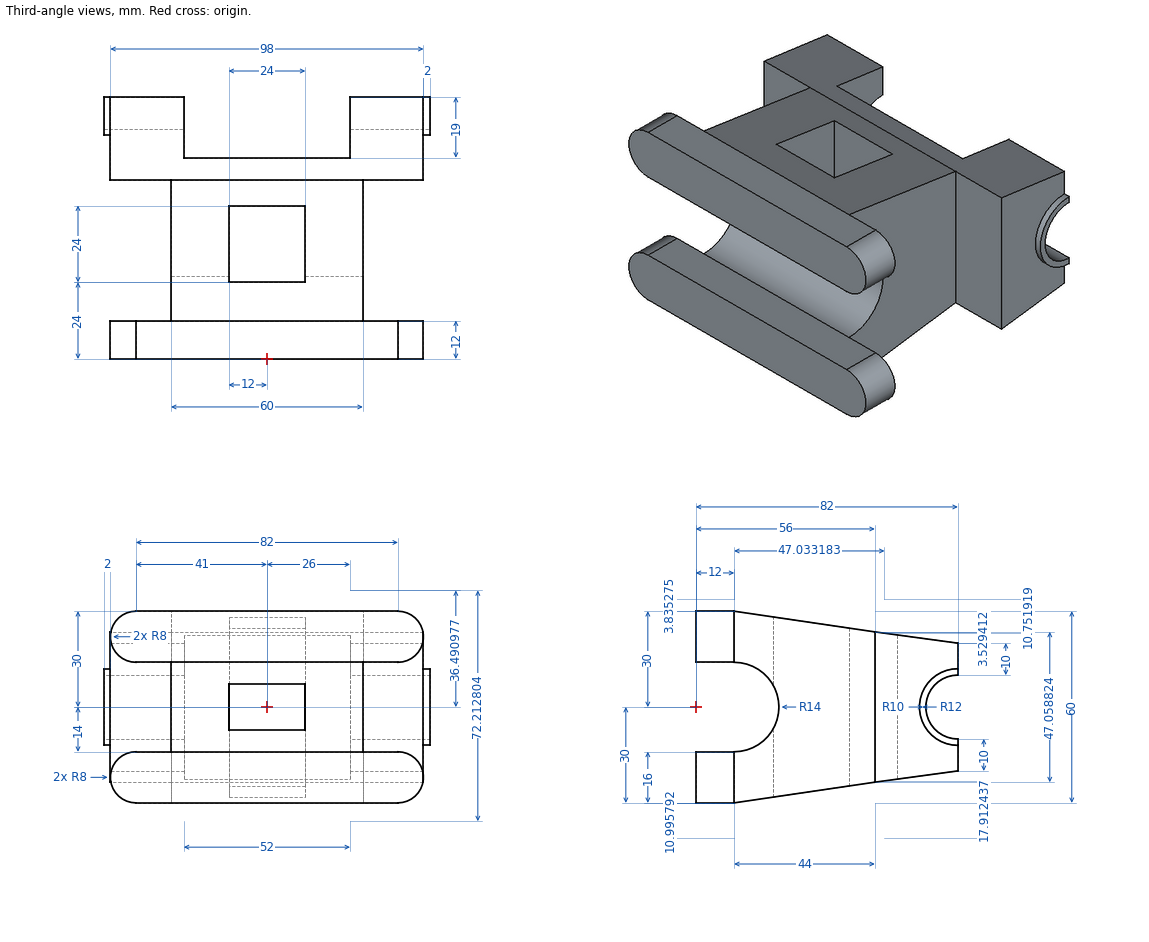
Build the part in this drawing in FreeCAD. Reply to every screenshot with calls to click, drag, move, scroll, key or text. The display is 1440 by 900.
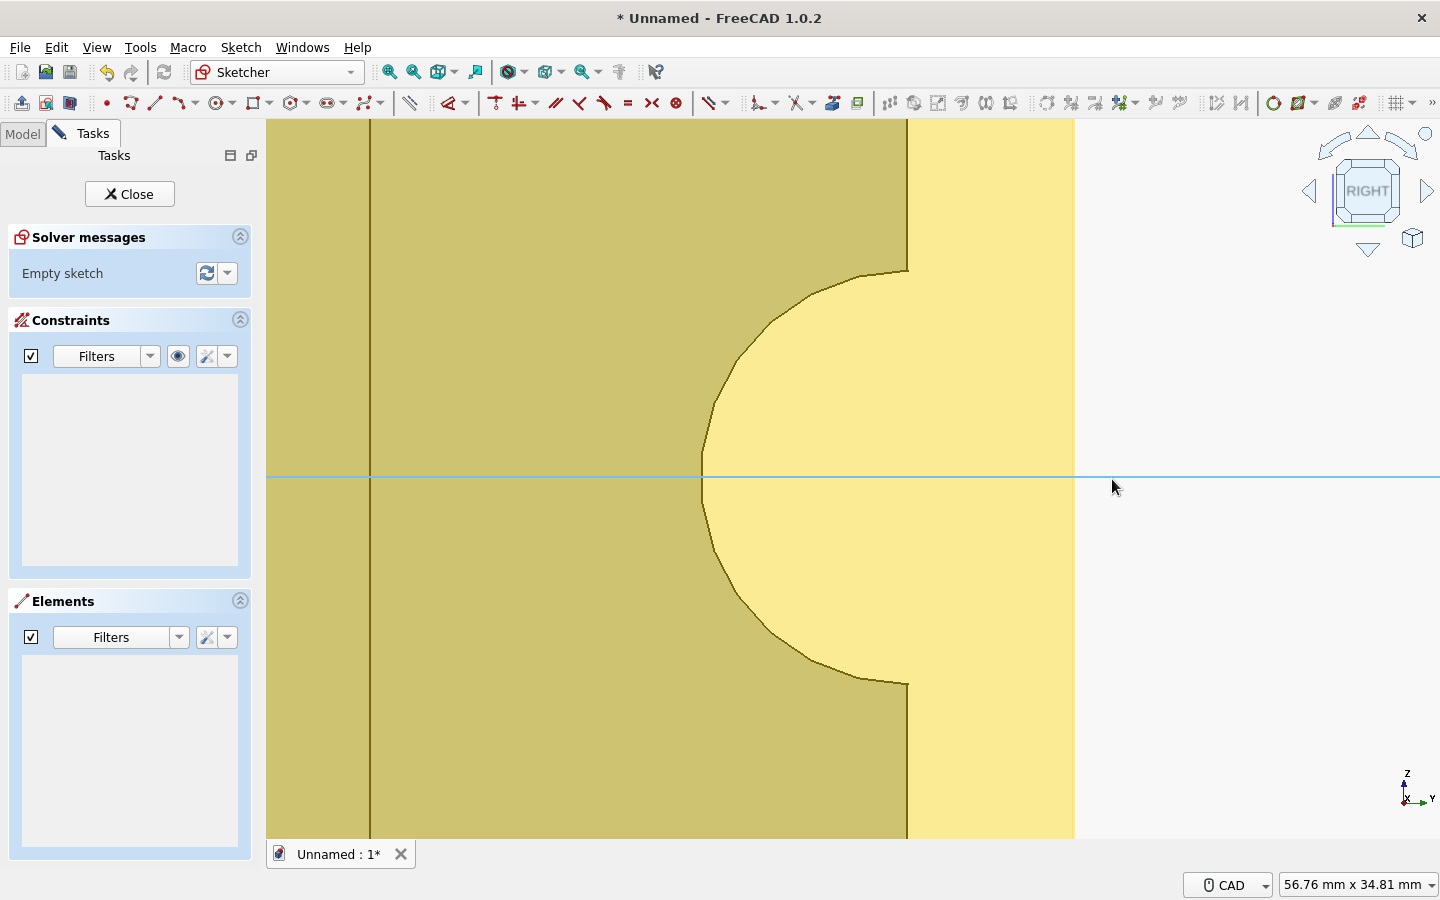
click(156, 104)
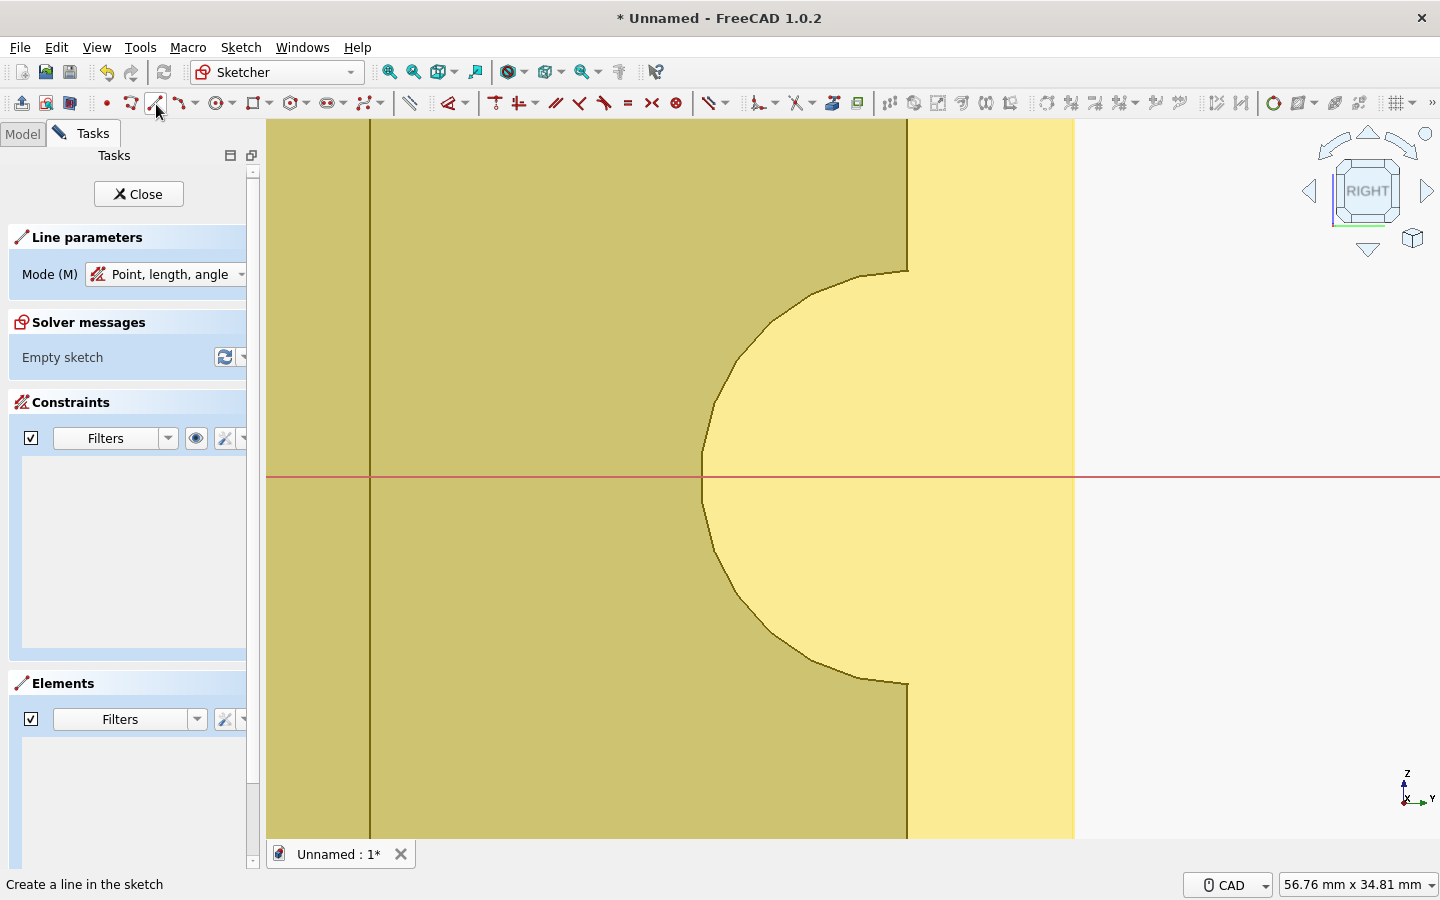
click(908, 271)
click(908, 229)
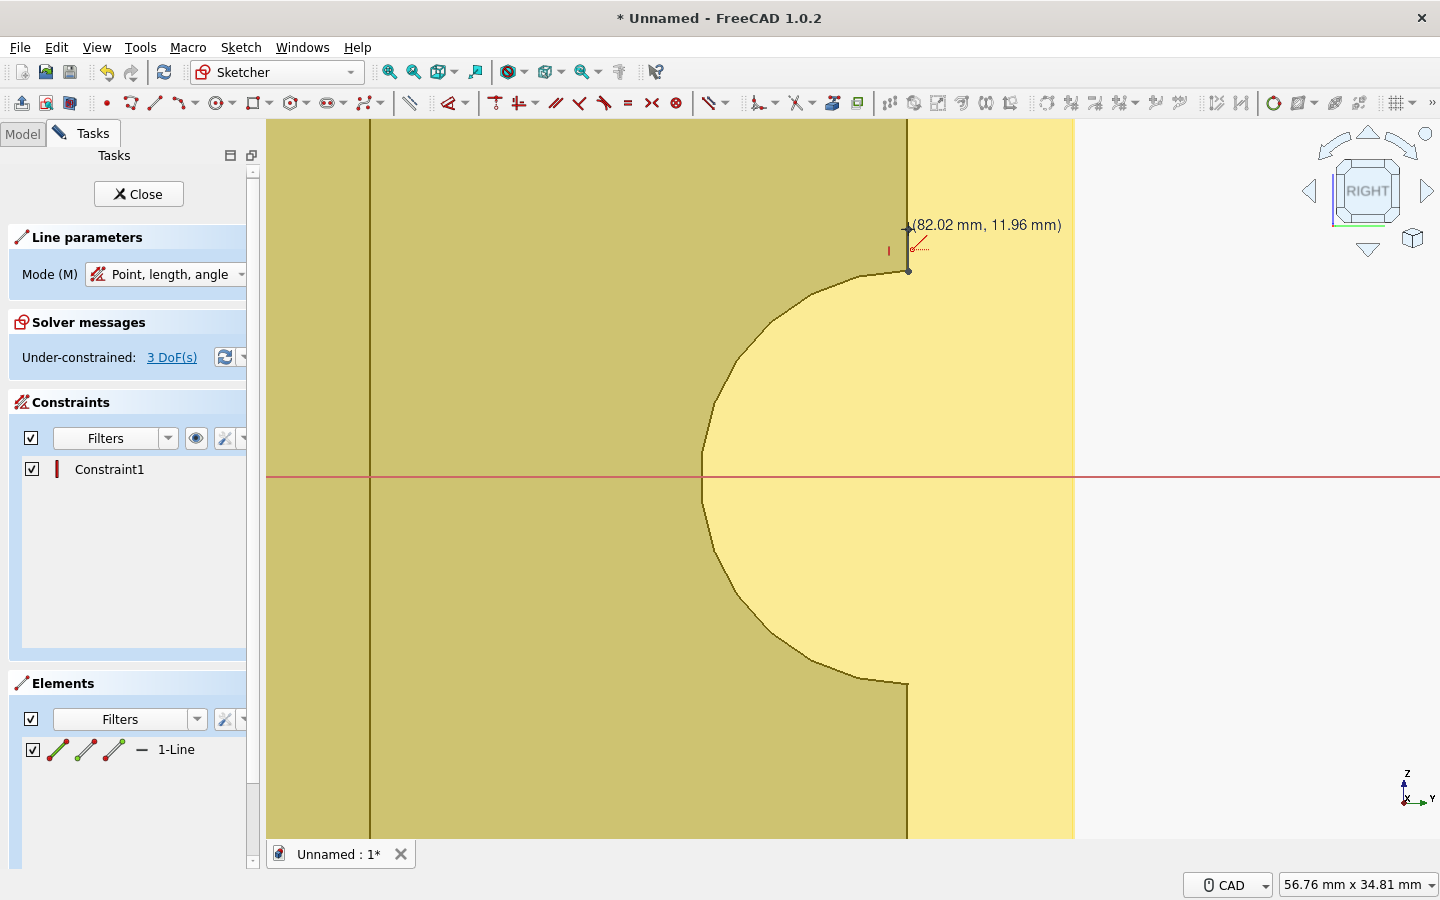
click(908, 726)
click(908, 684)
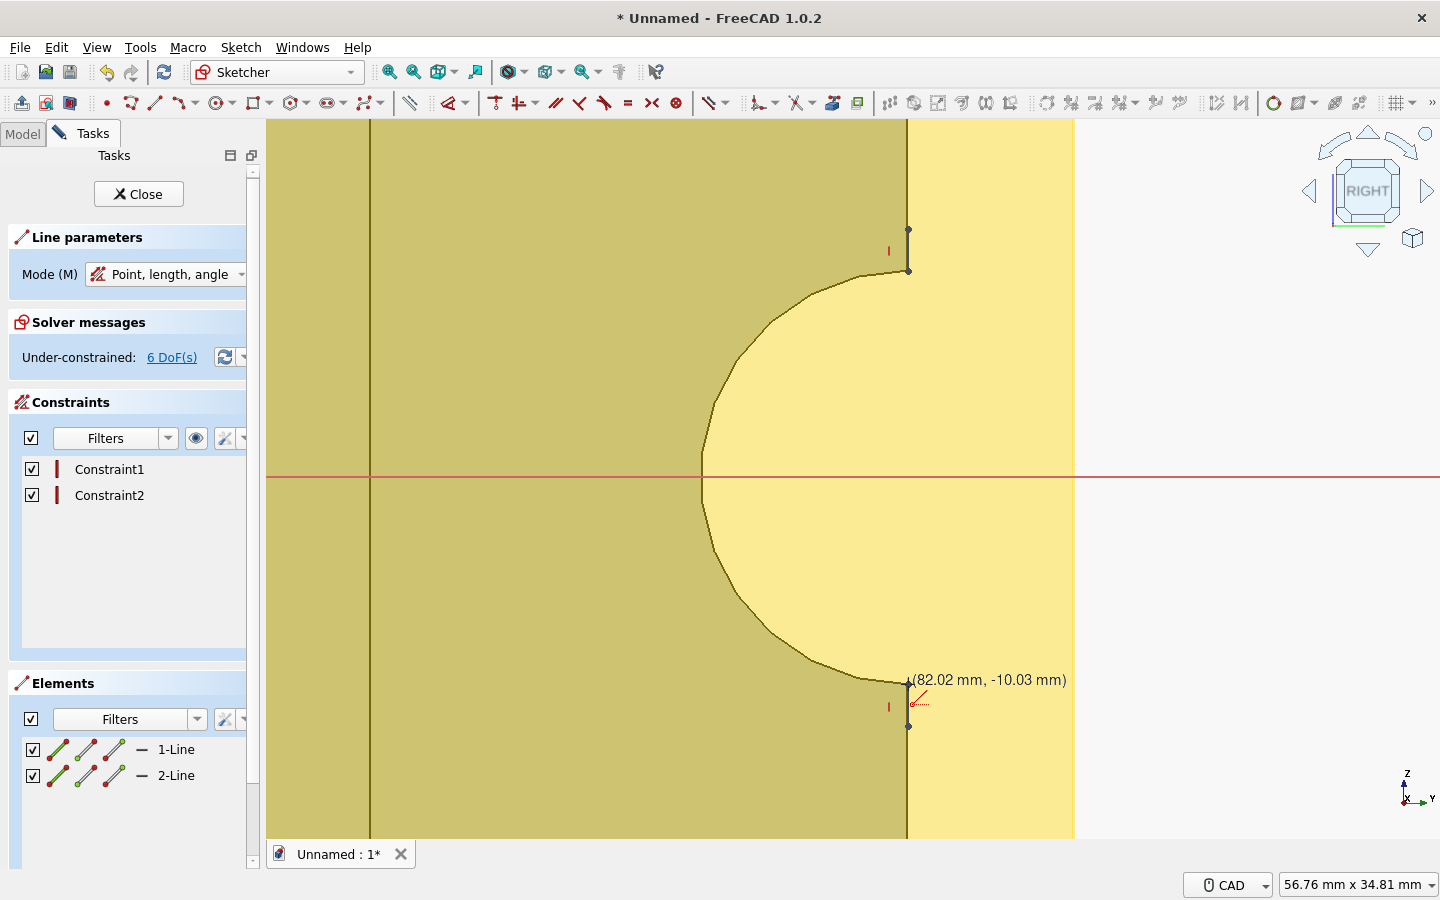
click(180, 104)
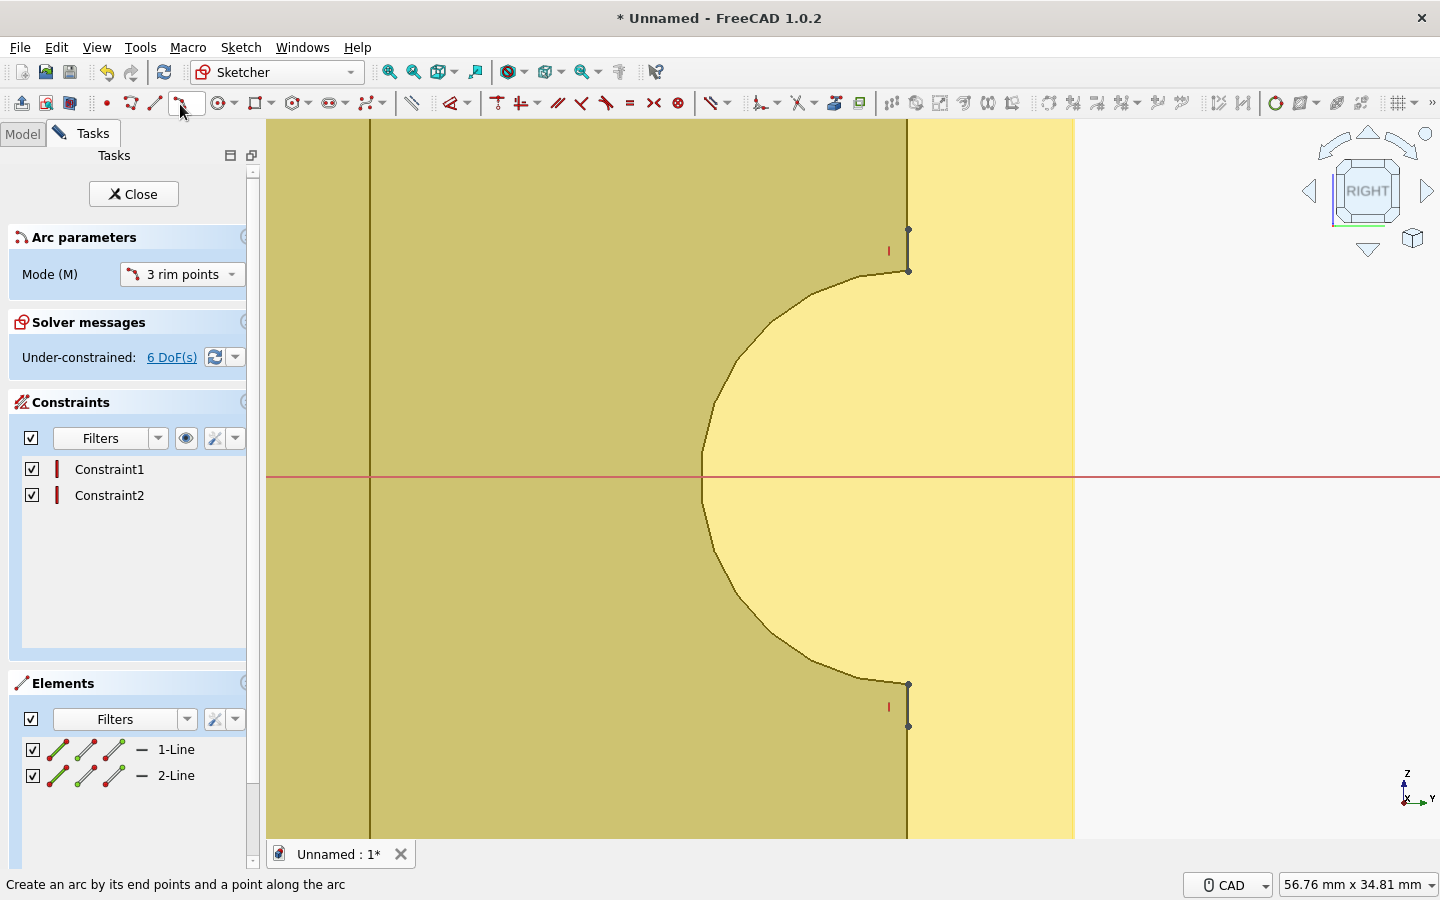
click(908, 230)
click(908, 727)
click(671, 401)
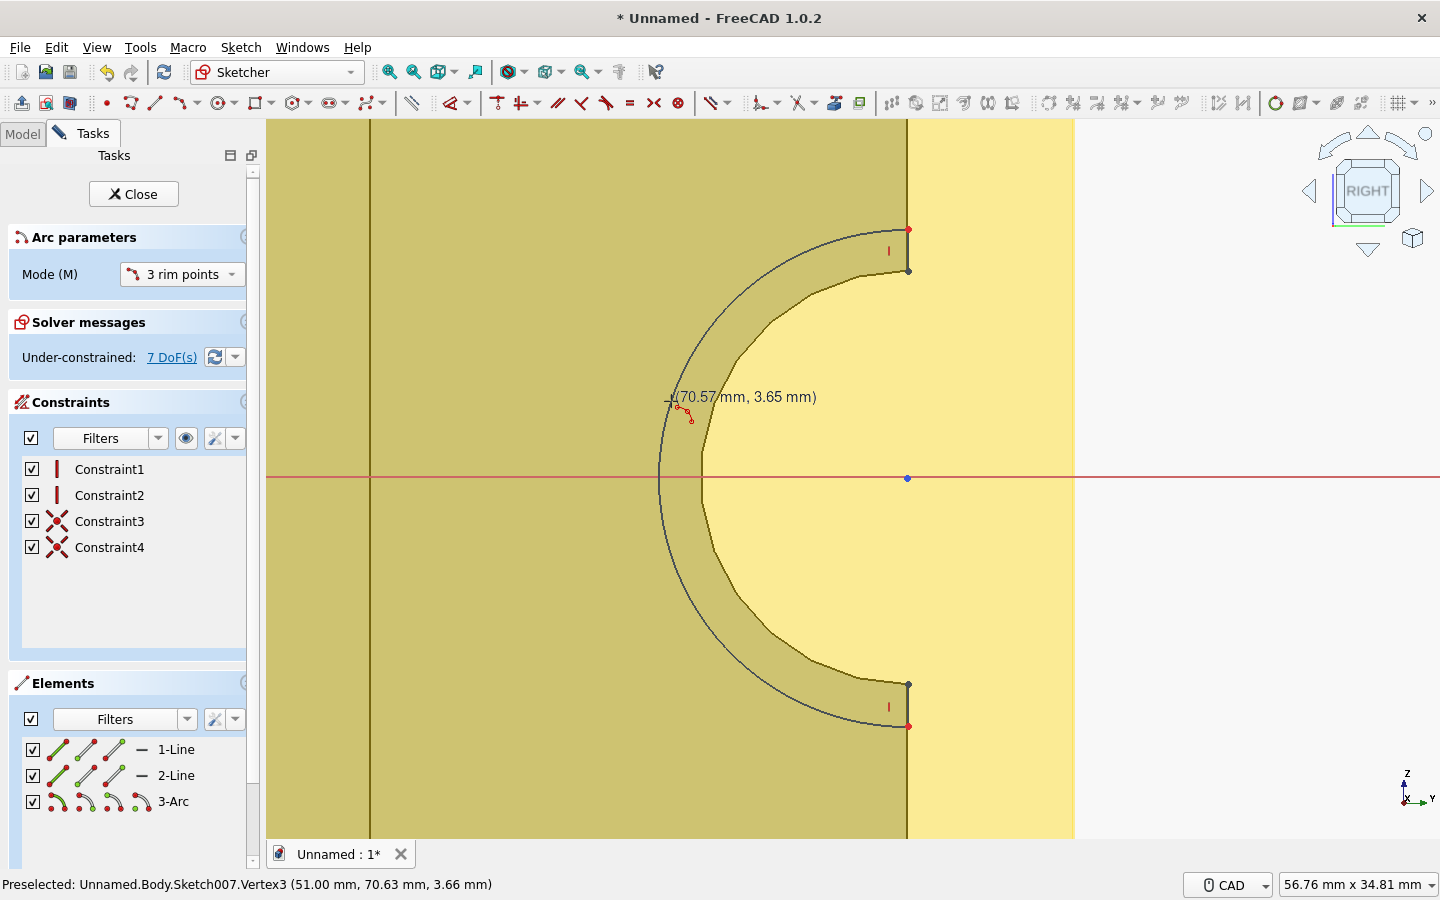
click(908, 685)
click(908, 272)
click(711, 414)
key(Escape)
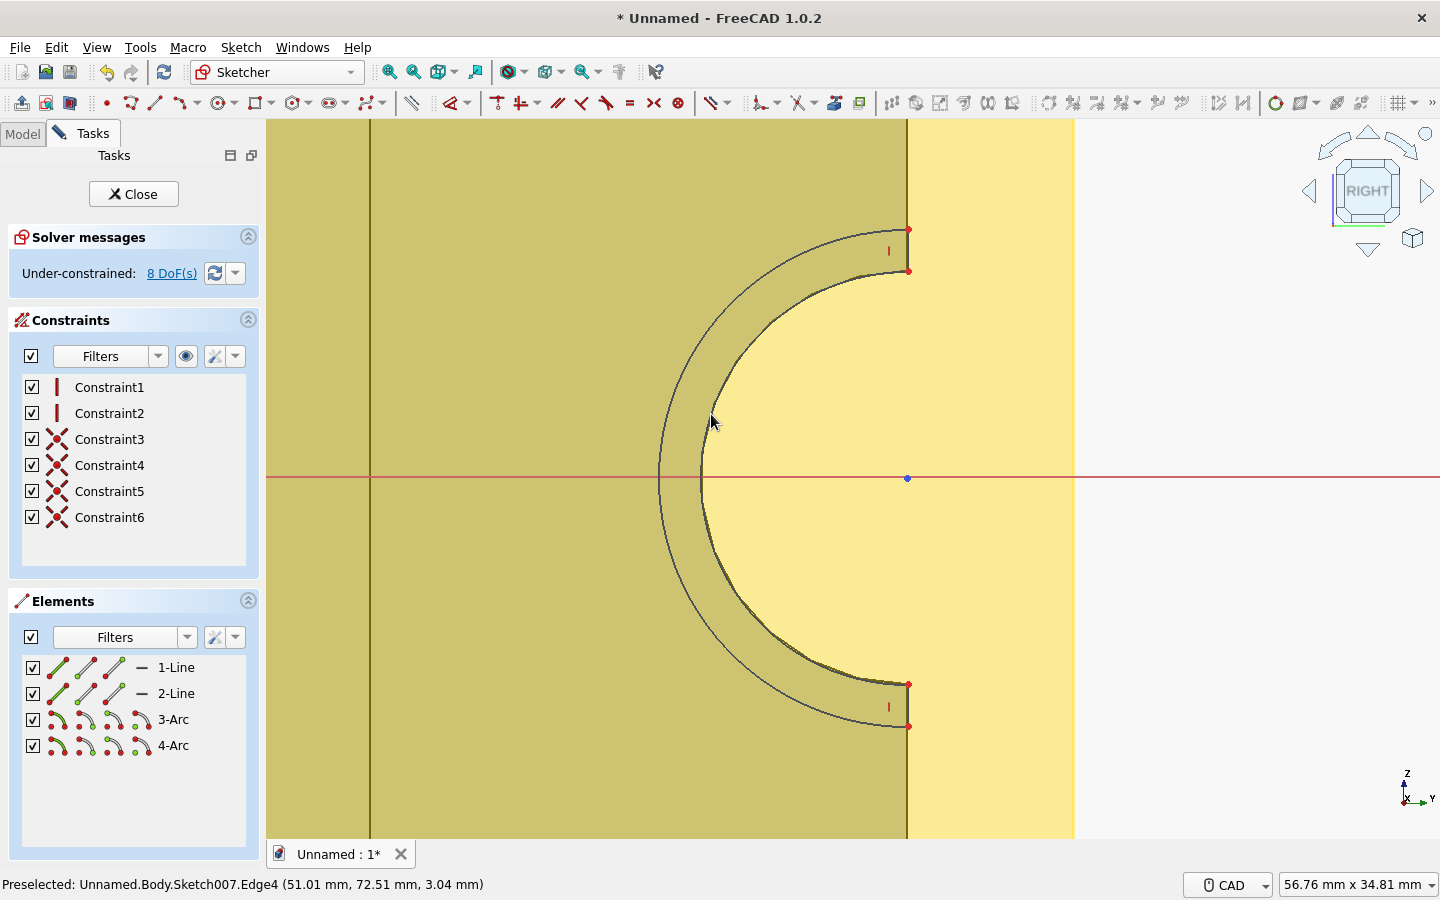
click(707, 332)